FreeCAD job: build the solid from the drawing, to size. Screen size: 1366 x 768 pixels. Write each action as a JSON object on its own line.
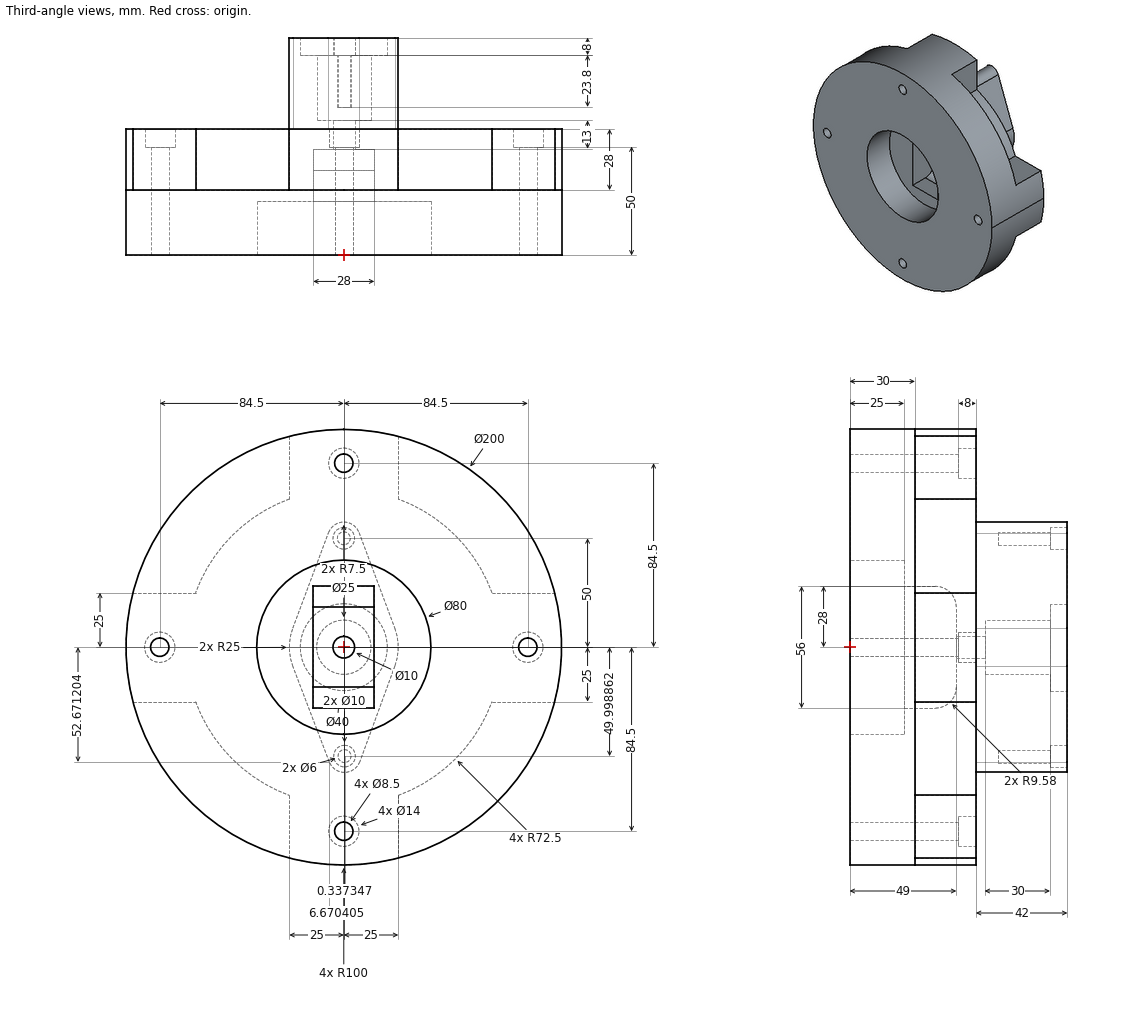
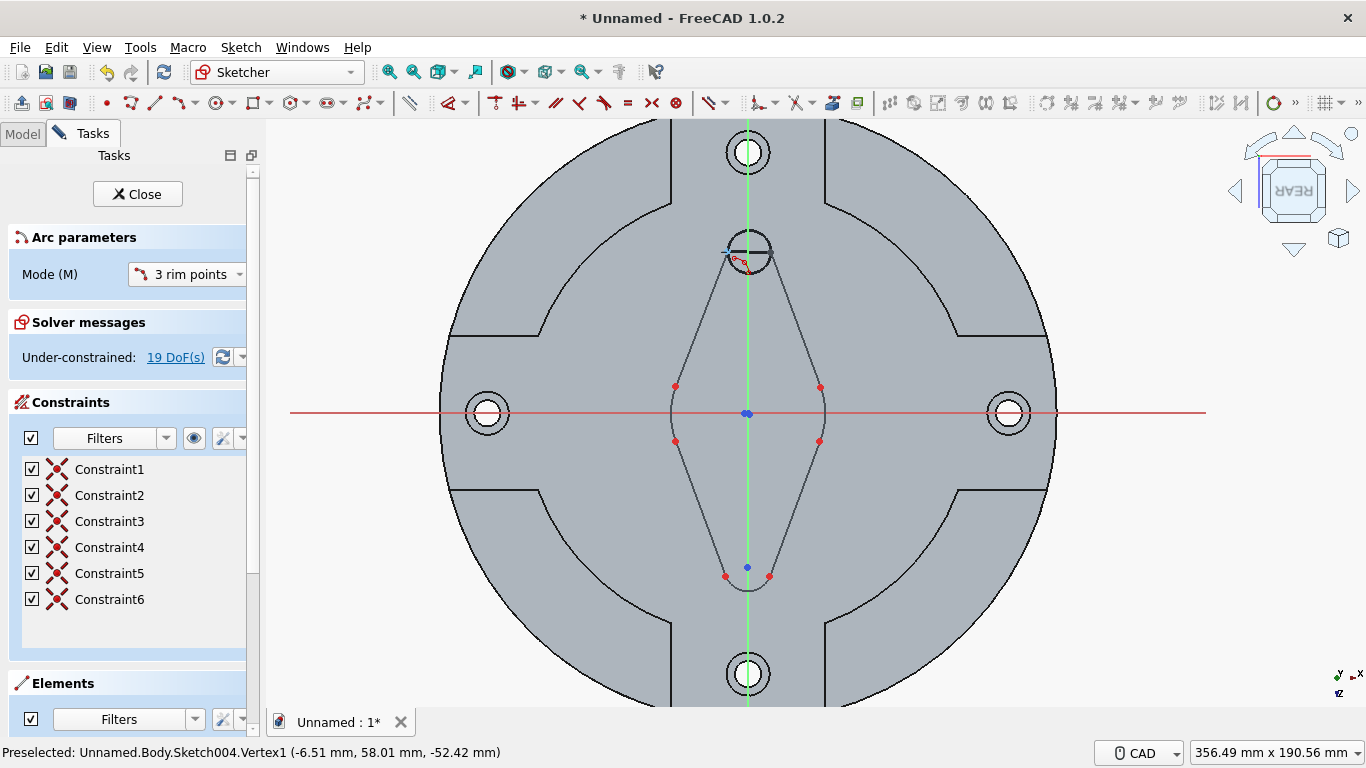
{"action": "scroll", "coordinate": [760, 239], "scroll_direction": "up", "scroll_amount": 2}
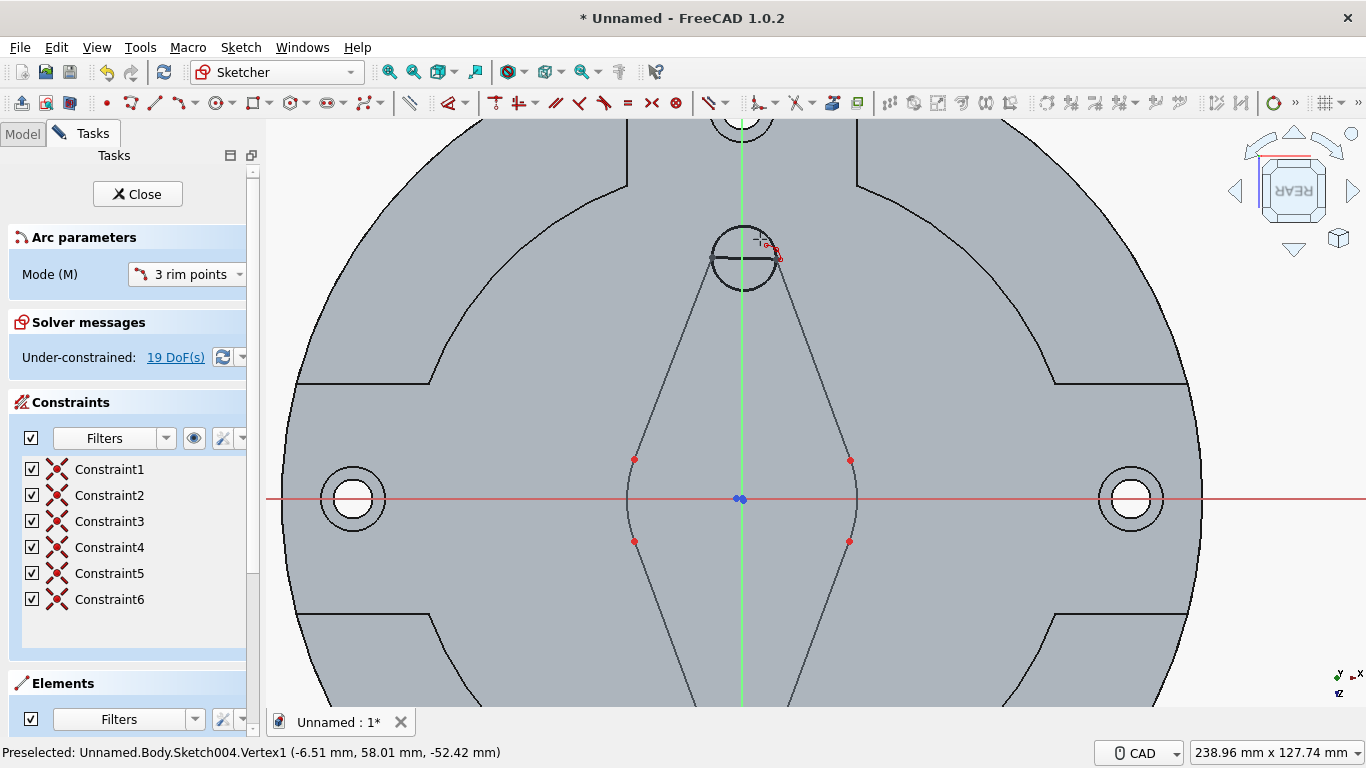
{"action": "left_click", "coordinate": [760, 238]}
{"action": "key", "text": "Escape"}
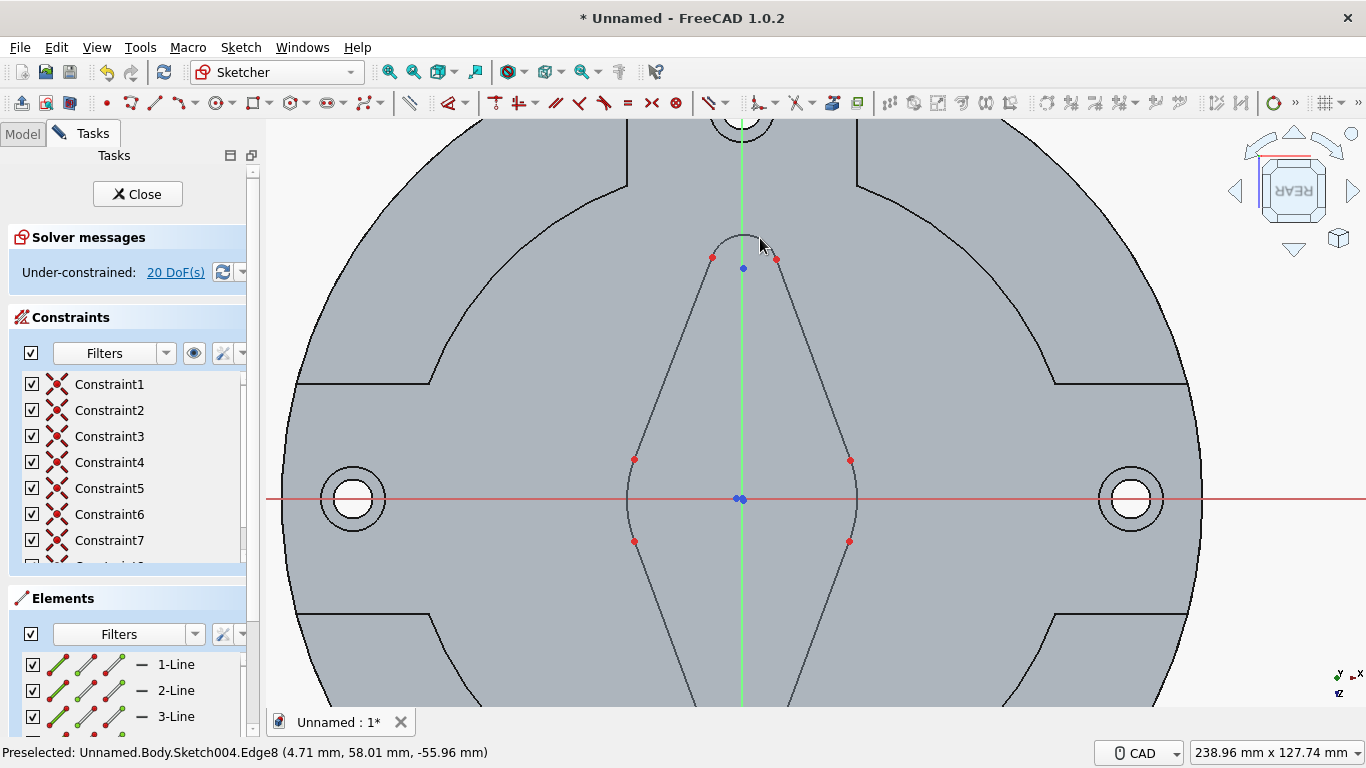
{"action": "left_click", "coordinate": [689, 318]}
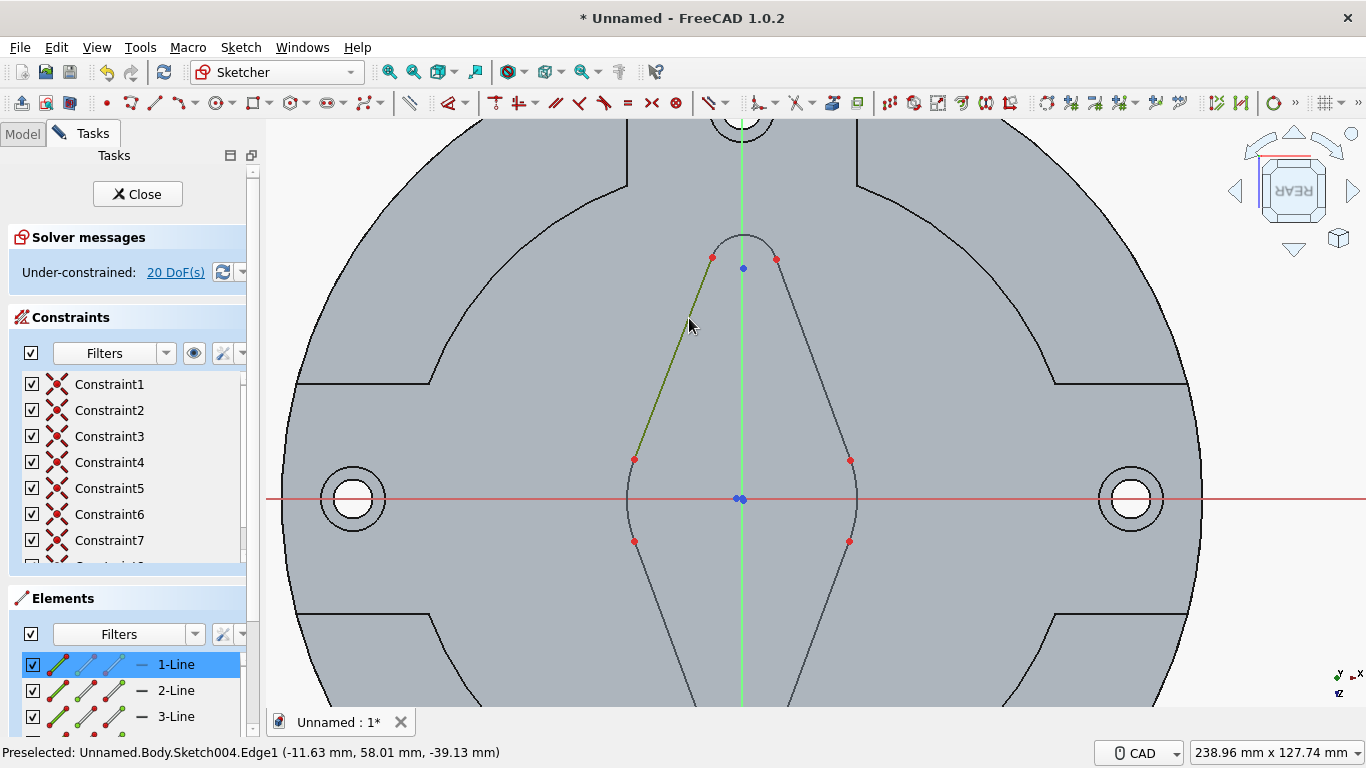
{"action": "left_click", "coordinate": [628, 483]}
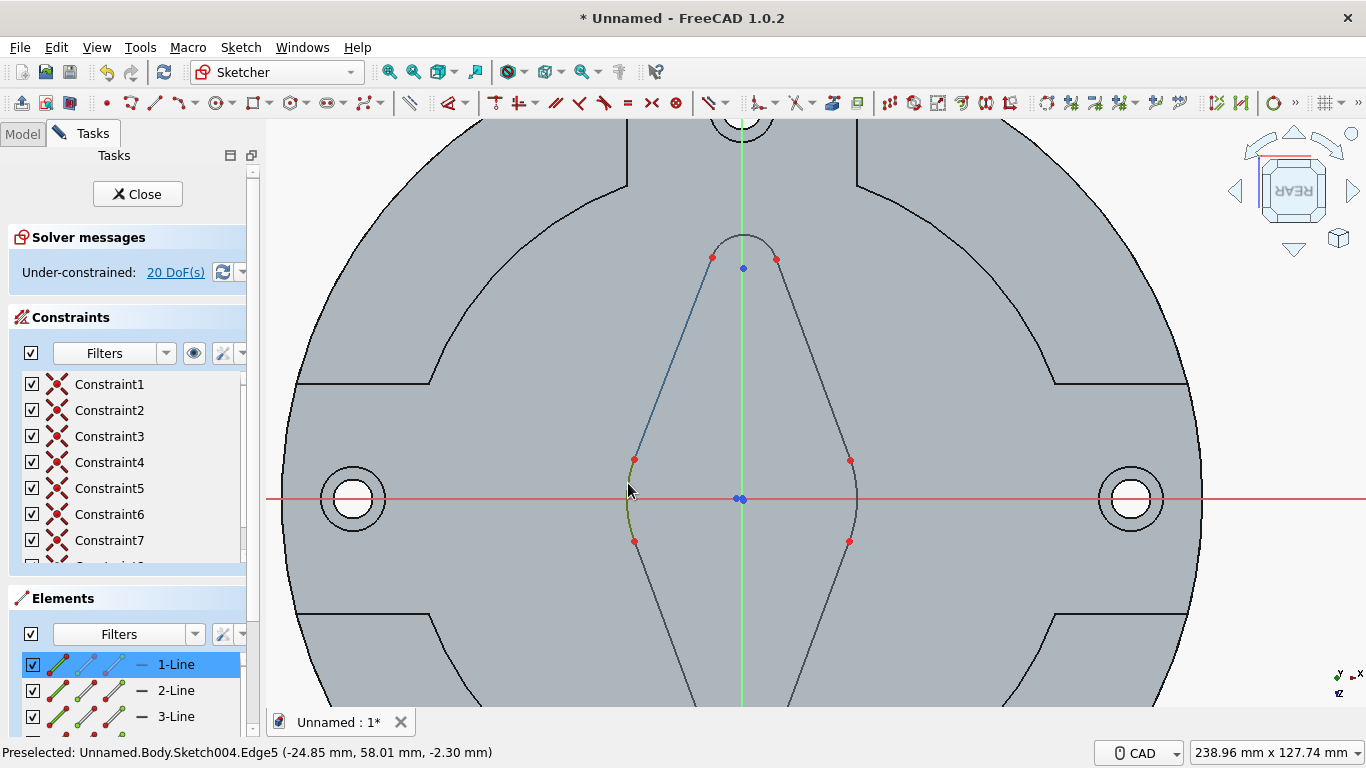
{"action": "key", "text": "t"}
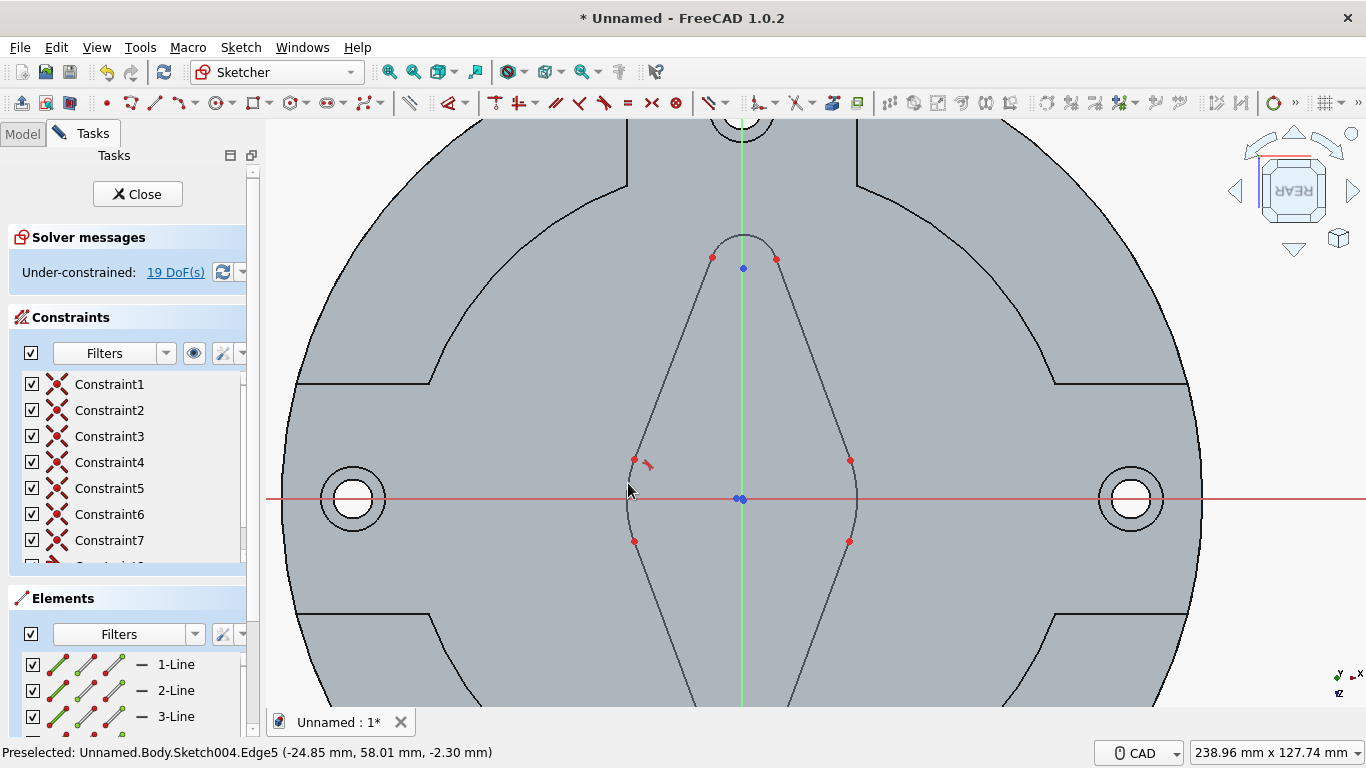
{"action": "left_click", "coordinate": [689, 318]}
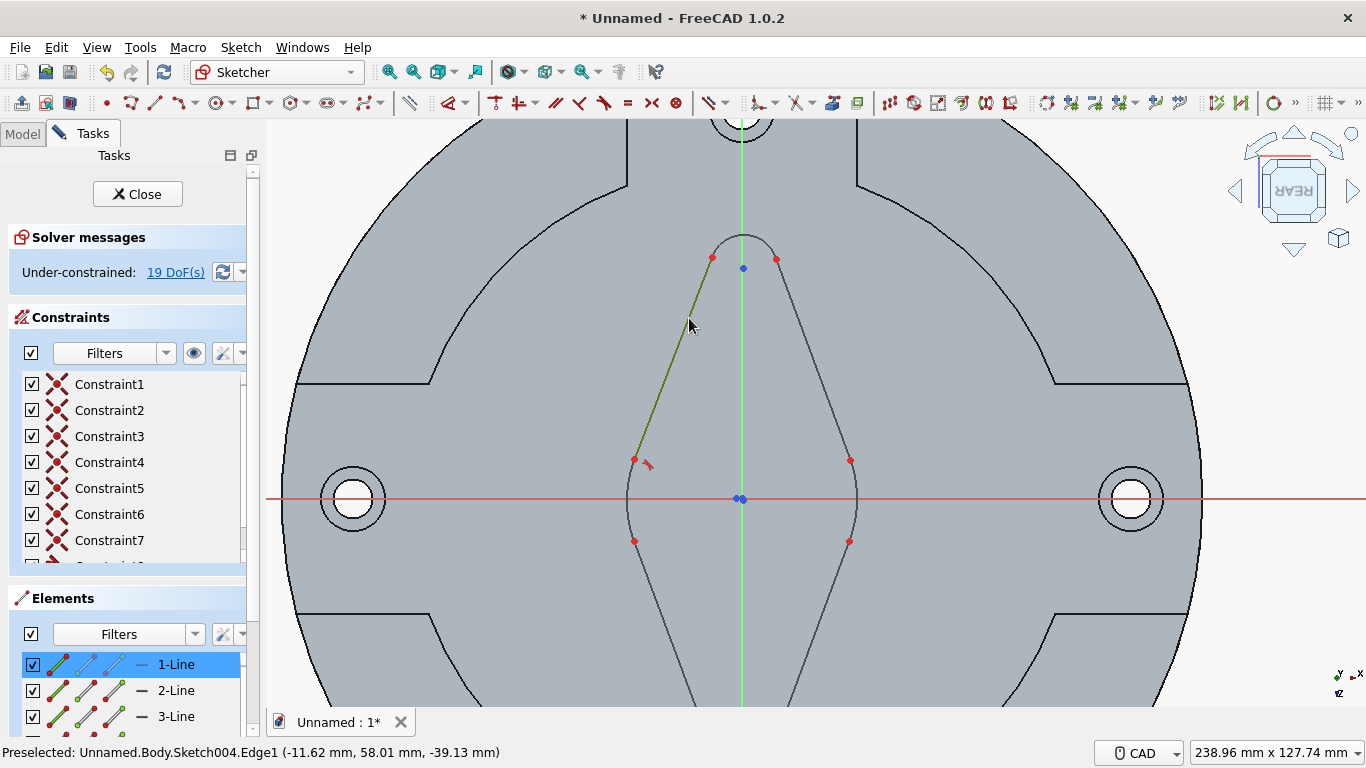
{"action": "left_click", "coordinate": [761, 239]}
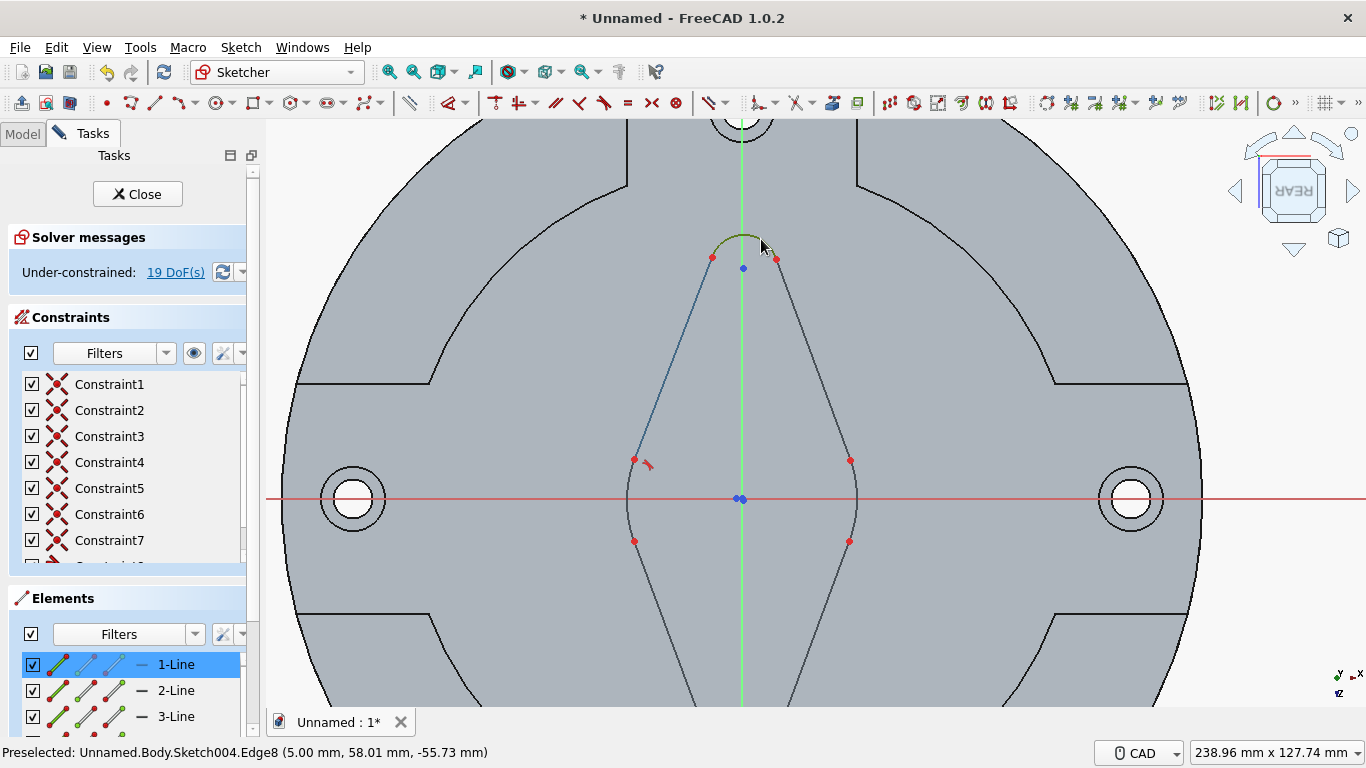
{"action": "key", "text": "t"}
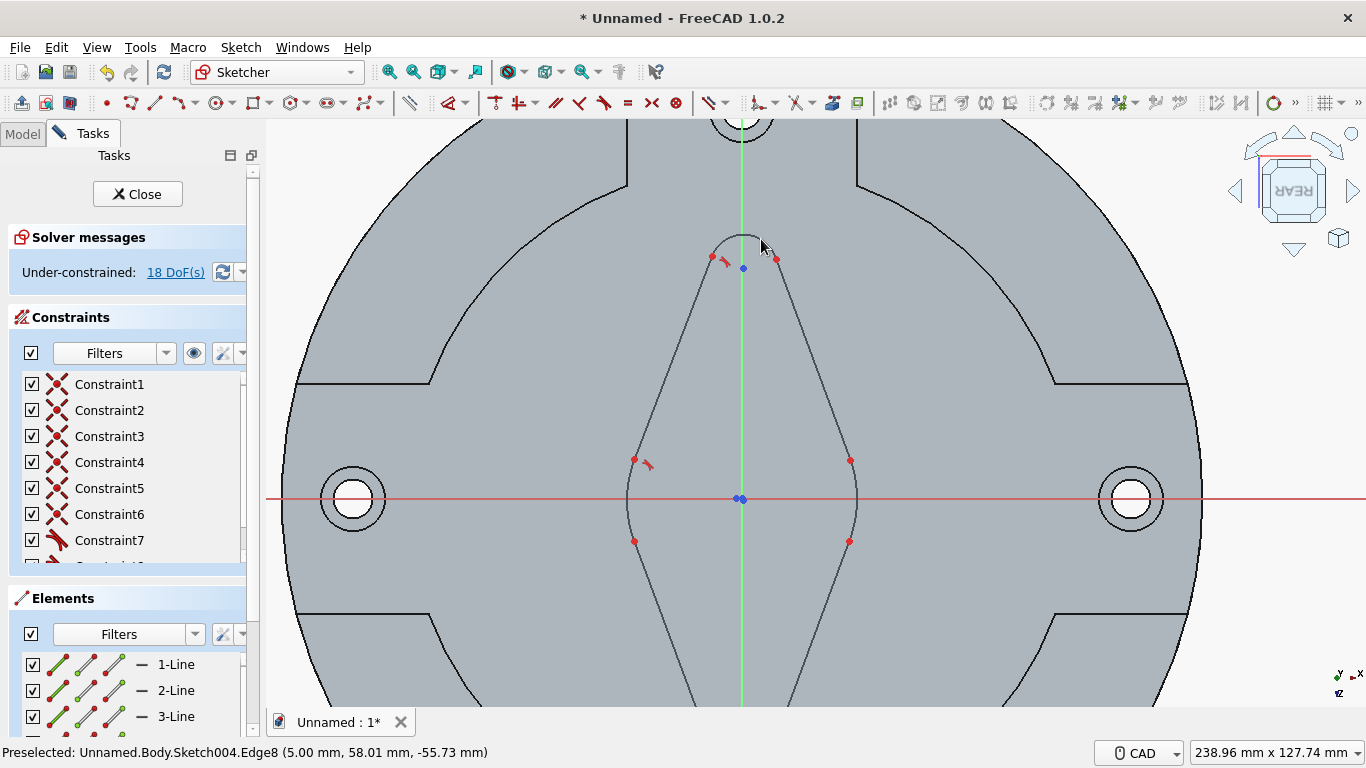
{"action": "left_click", "coordinate": [657, 601]}